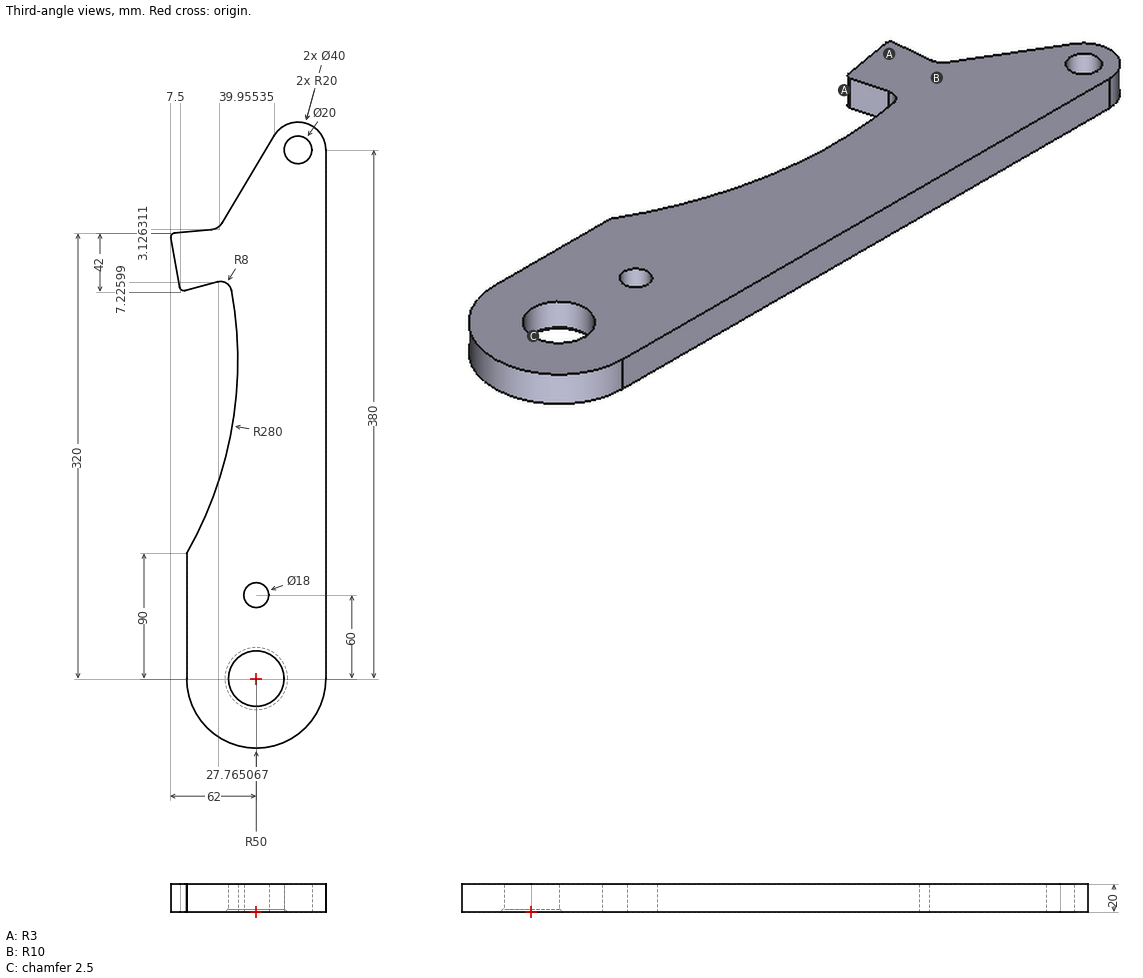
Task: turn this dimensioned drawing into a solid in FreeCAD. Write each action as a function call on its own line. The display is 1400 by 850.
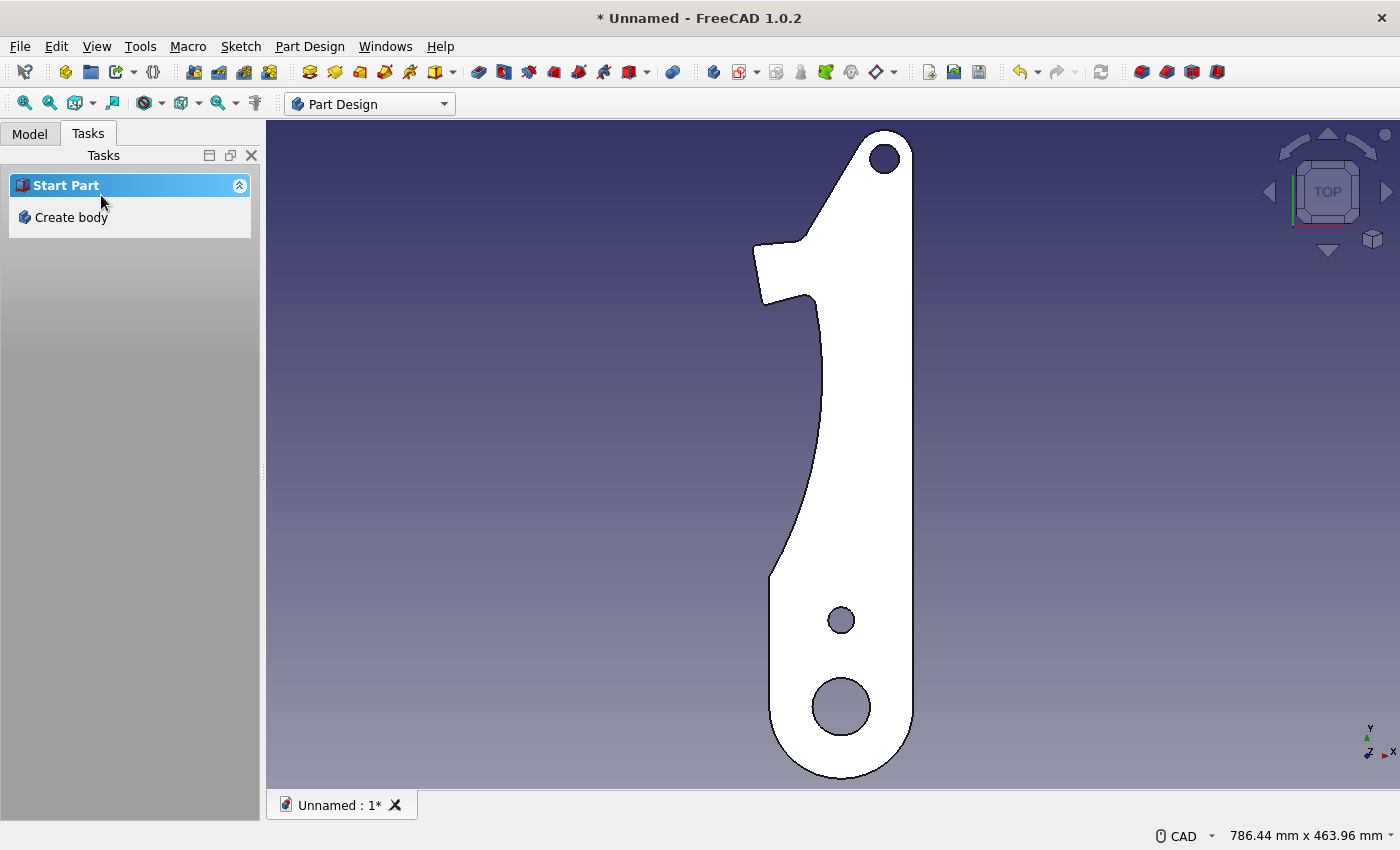
key(0)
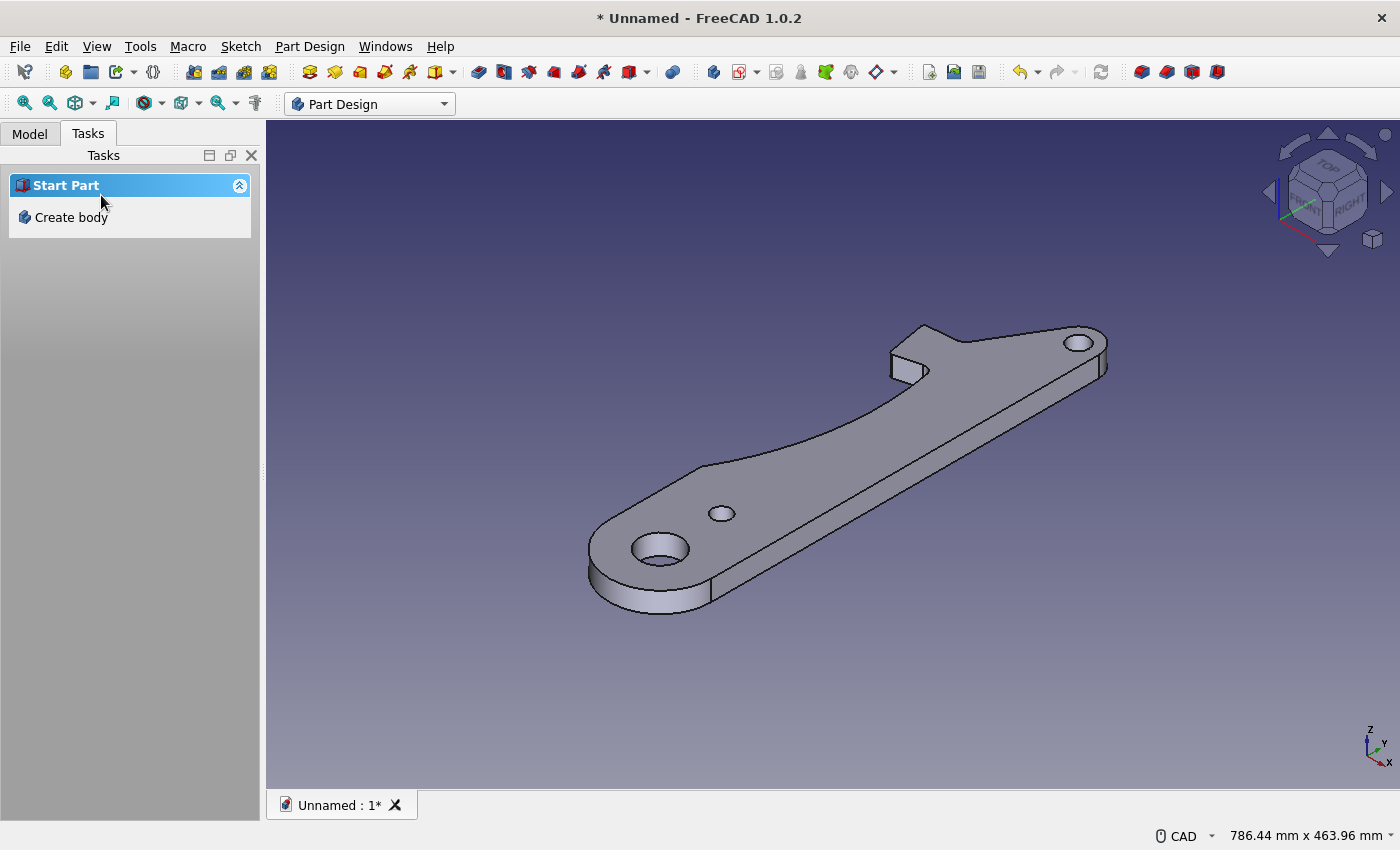
key(1)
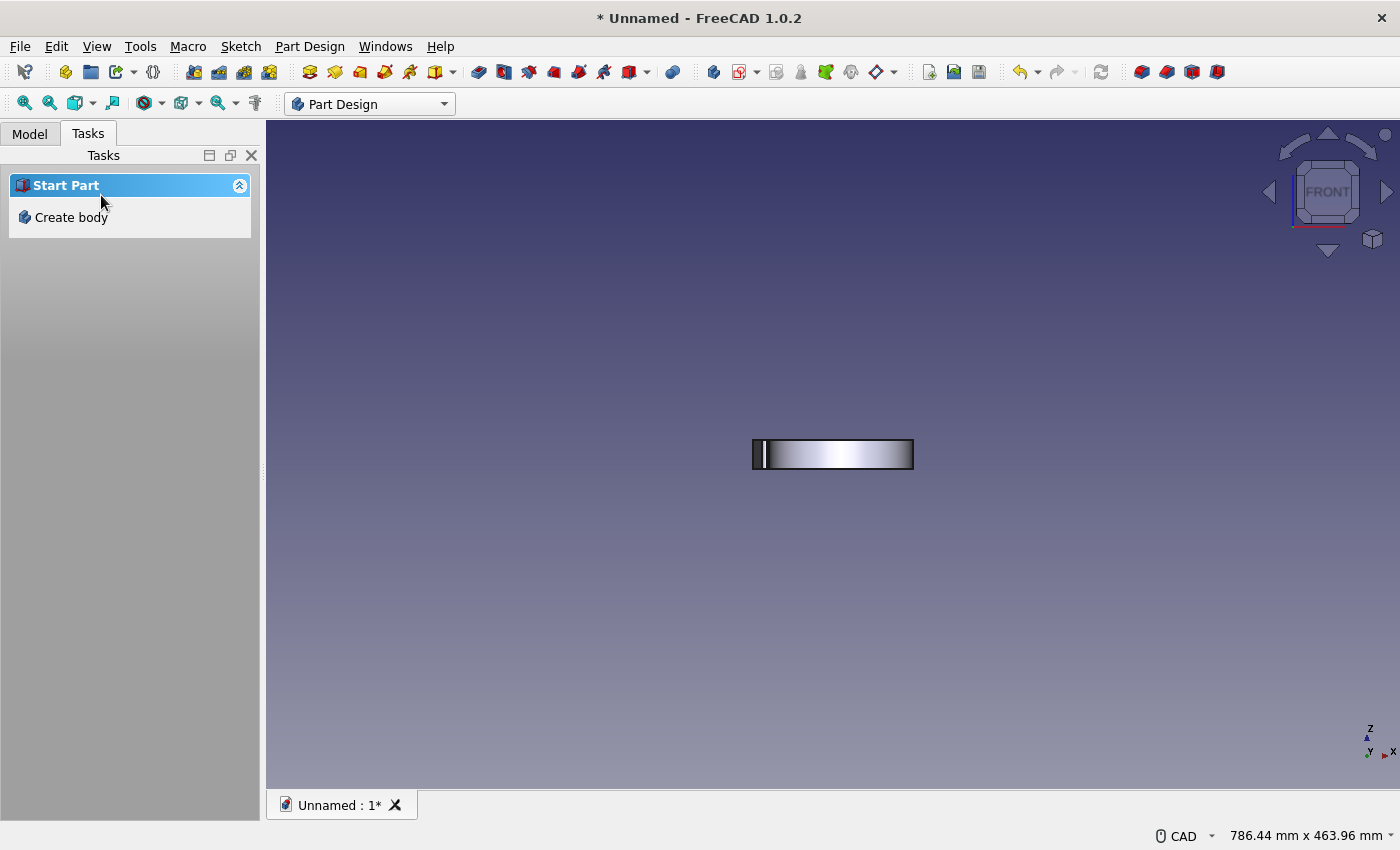
click(25, 104)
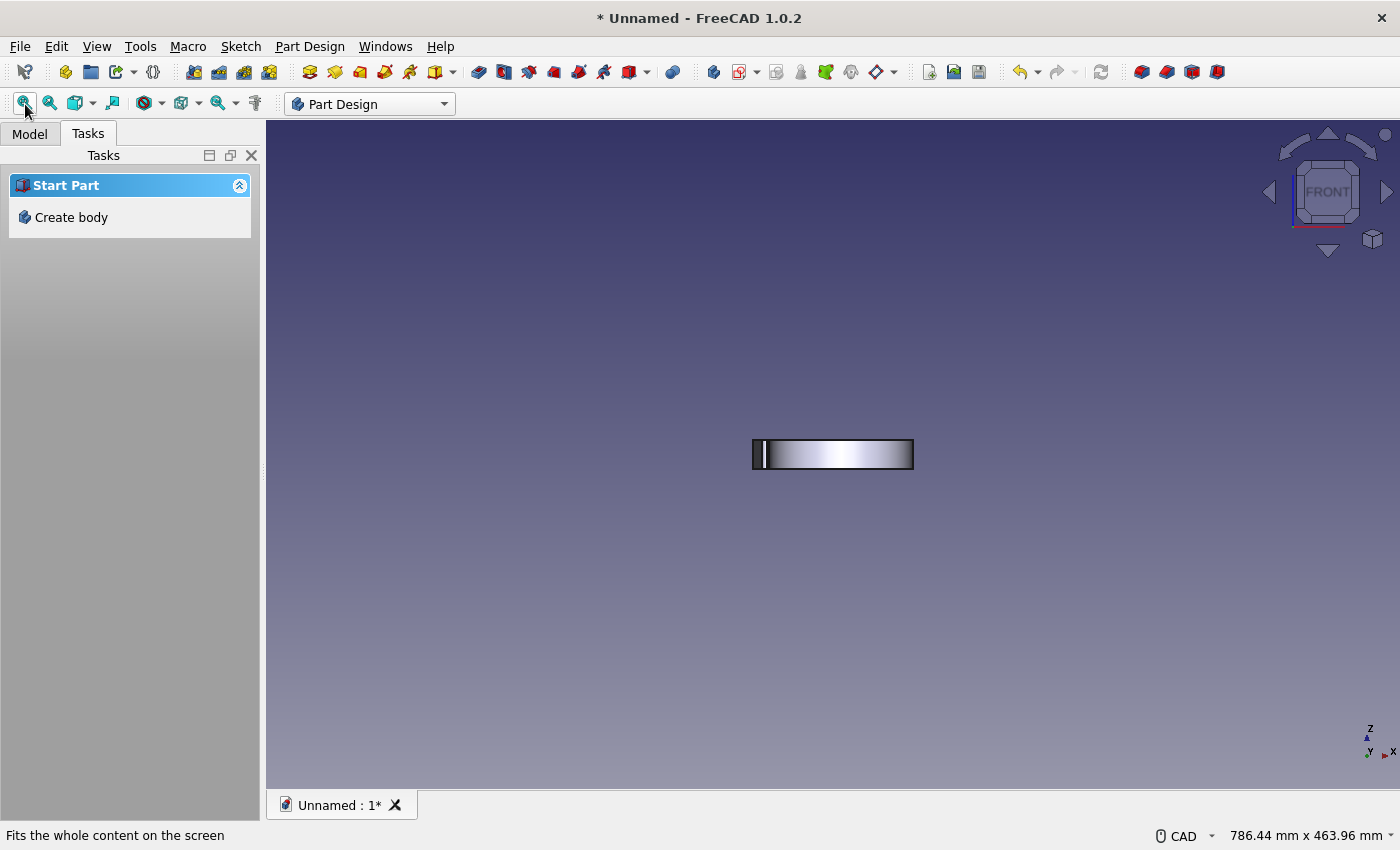
key(3)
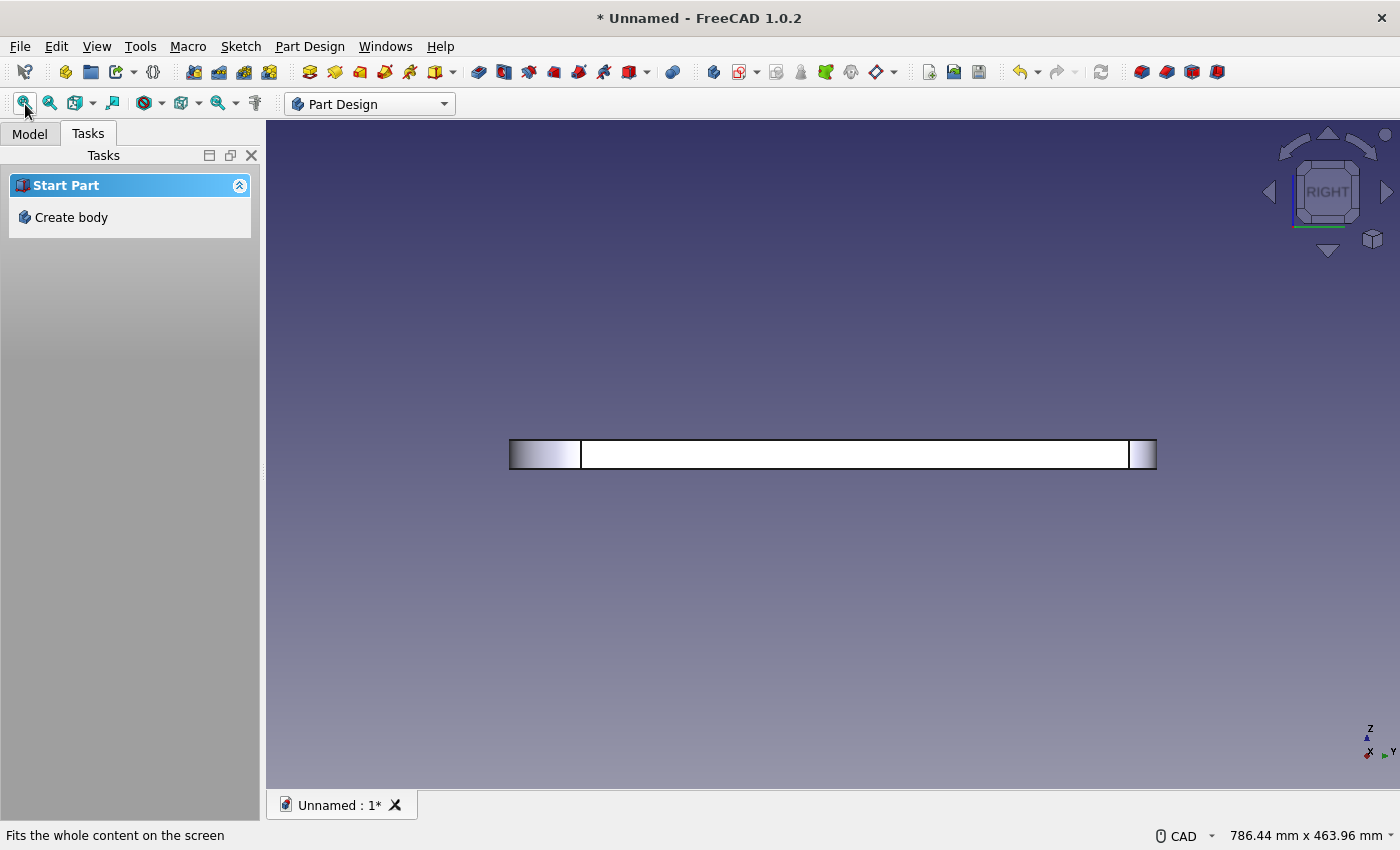
key(5)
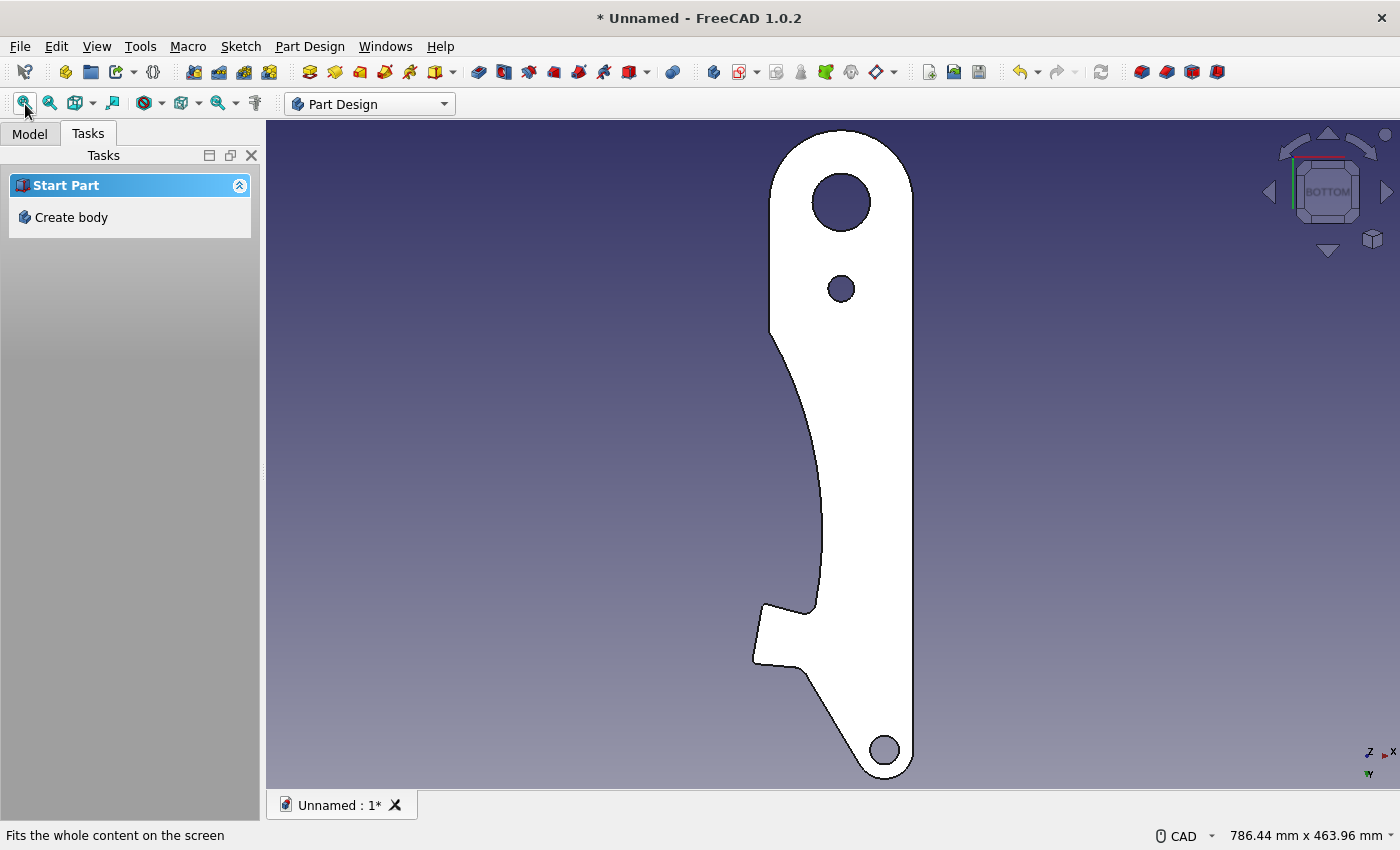
click(818, 184)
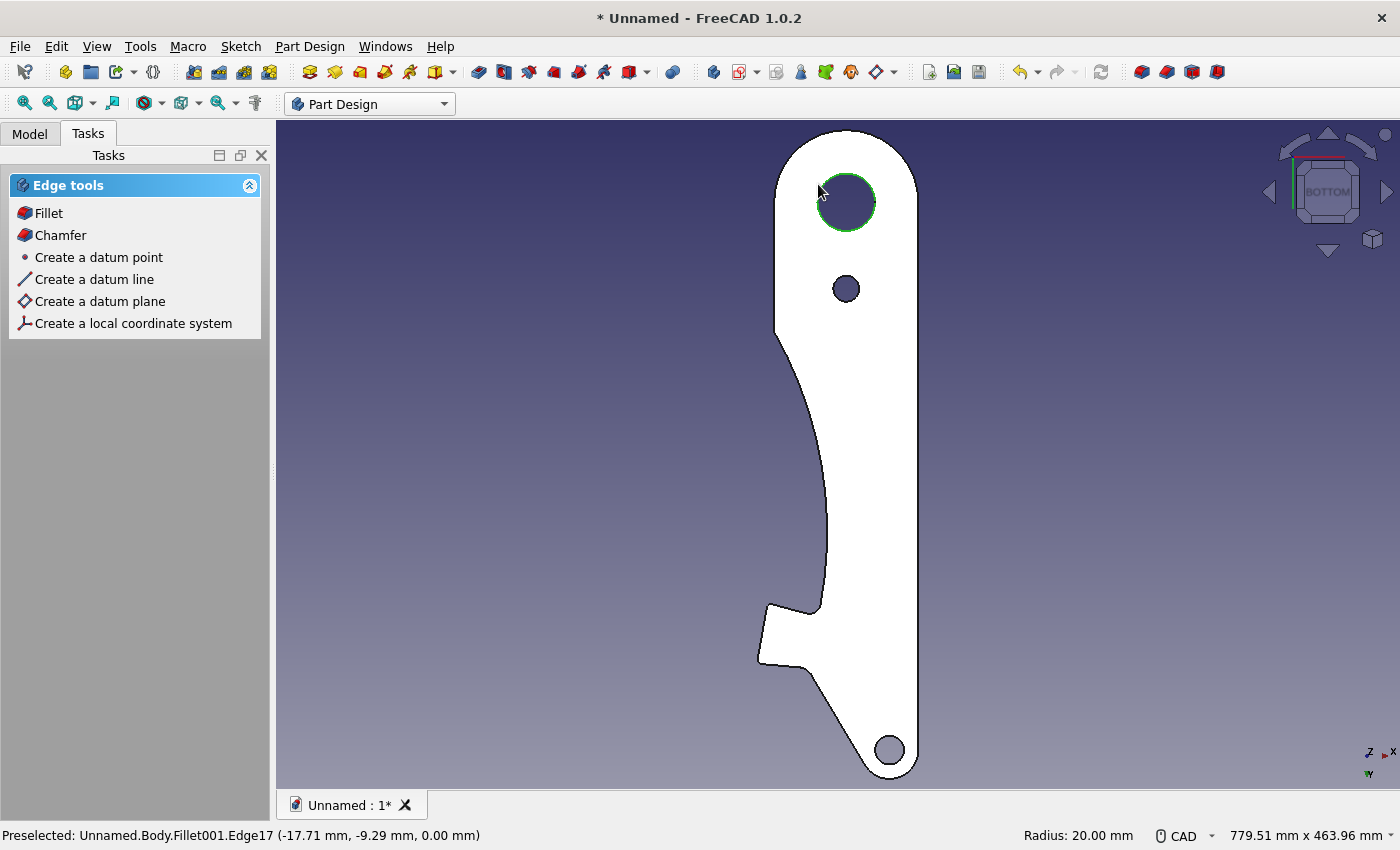
click(1167, 72)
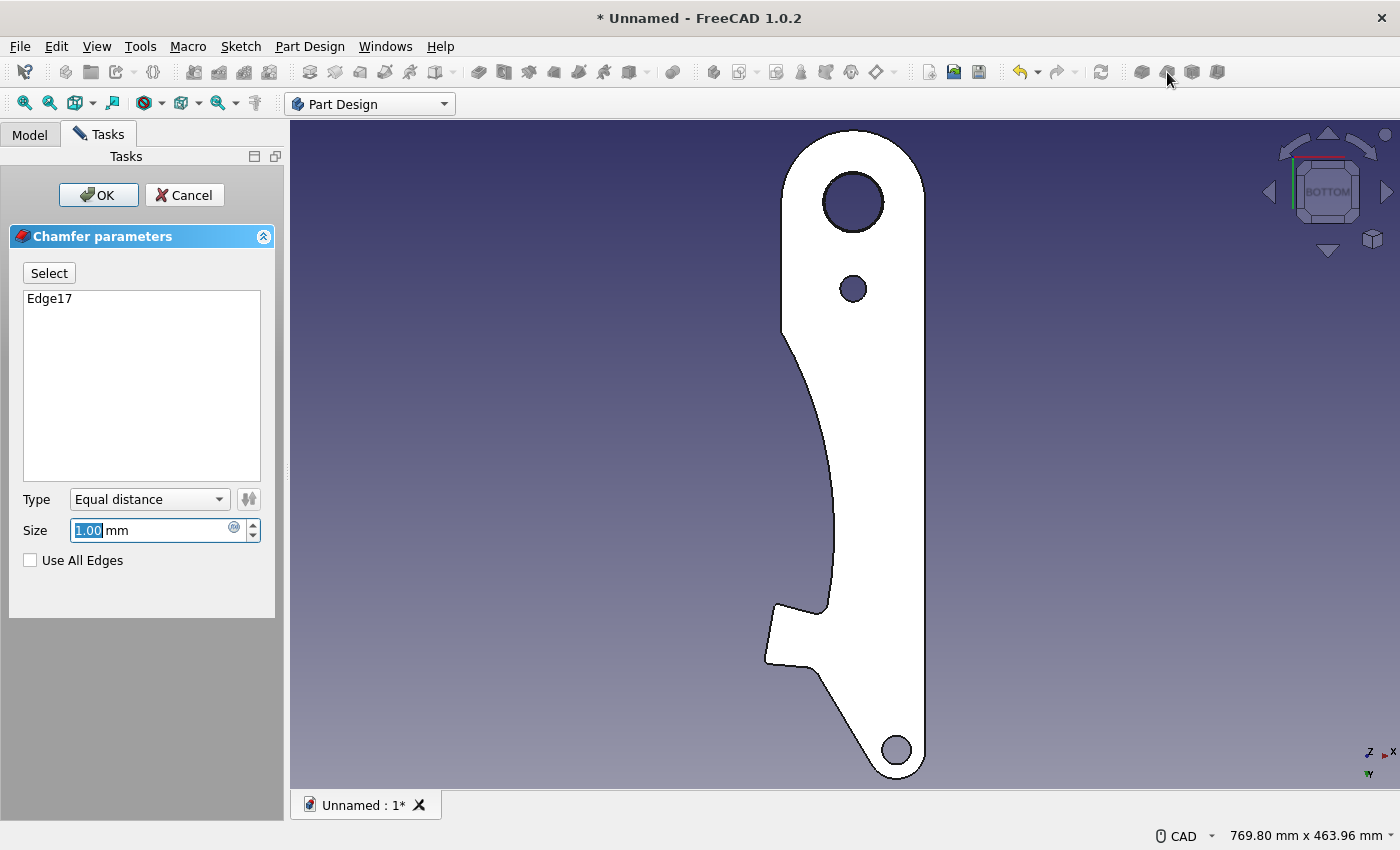
text(2.5)
key(Tab)